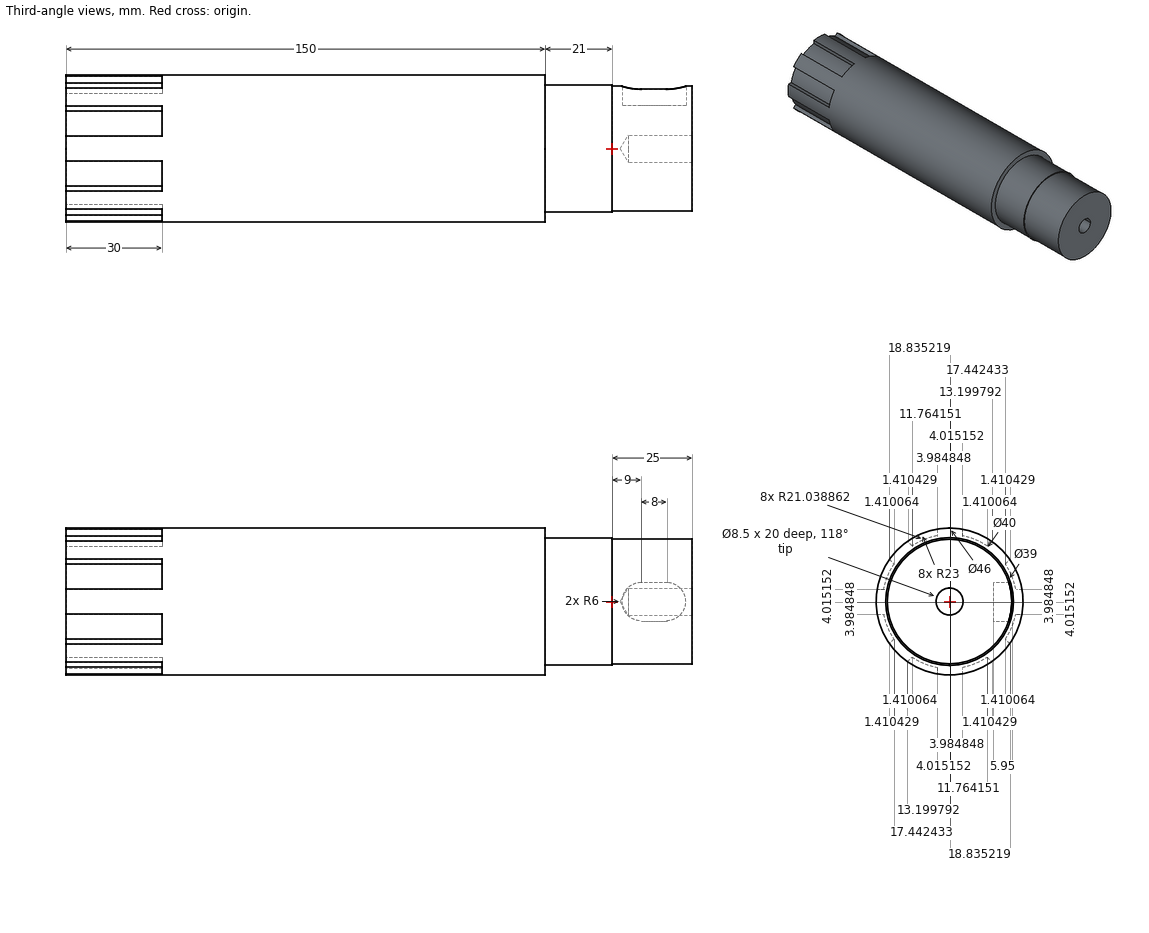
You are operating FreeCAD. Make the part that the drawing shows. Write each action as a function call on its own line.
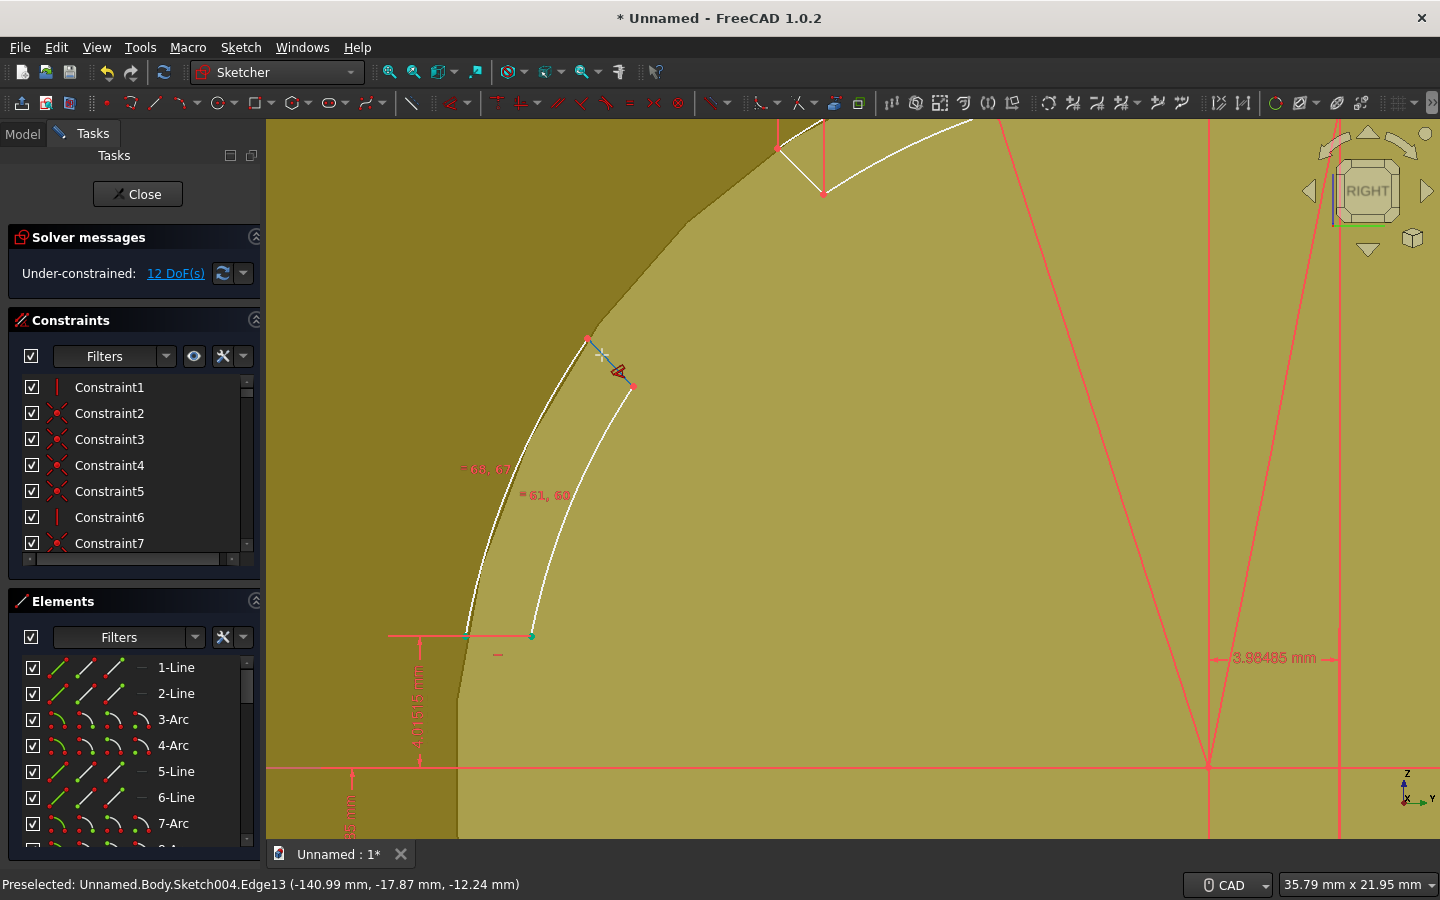
click(602, 353)
click(611, 305)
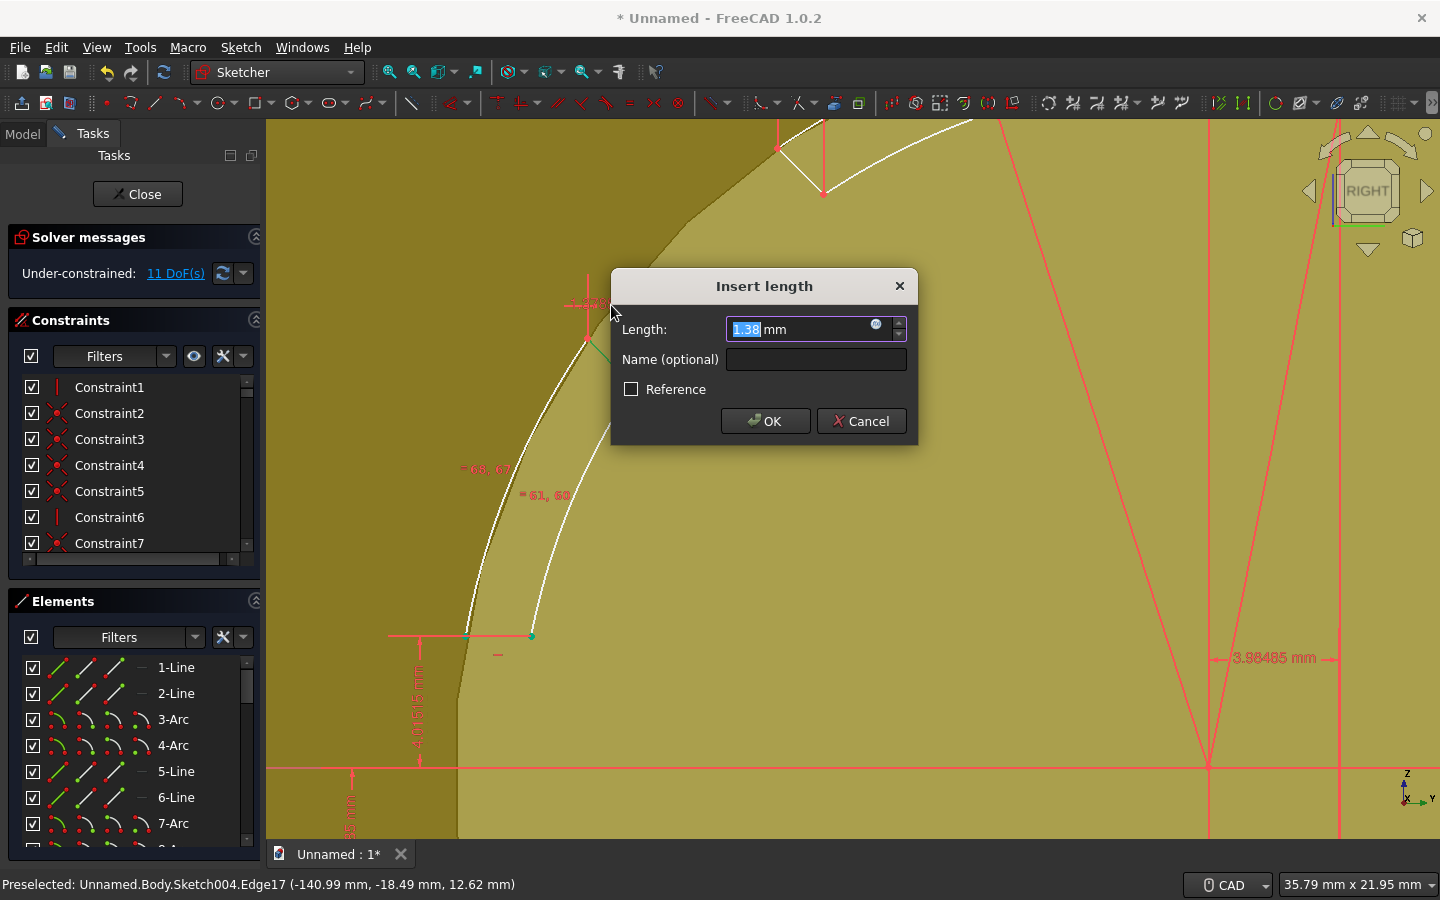
text(1.410064)
key(Return)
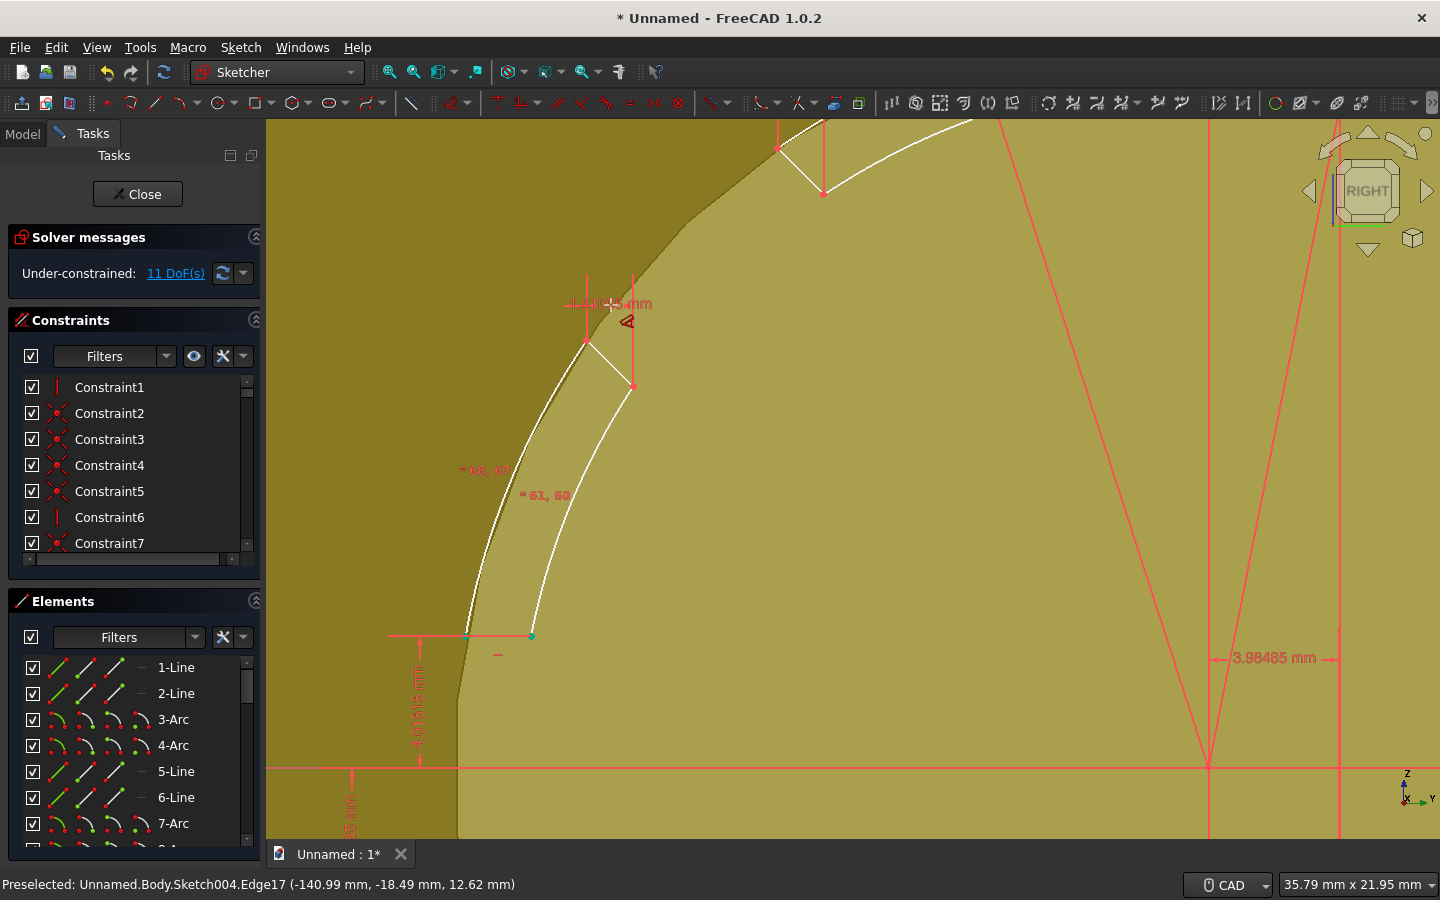
scroll(602, 355, down, 6)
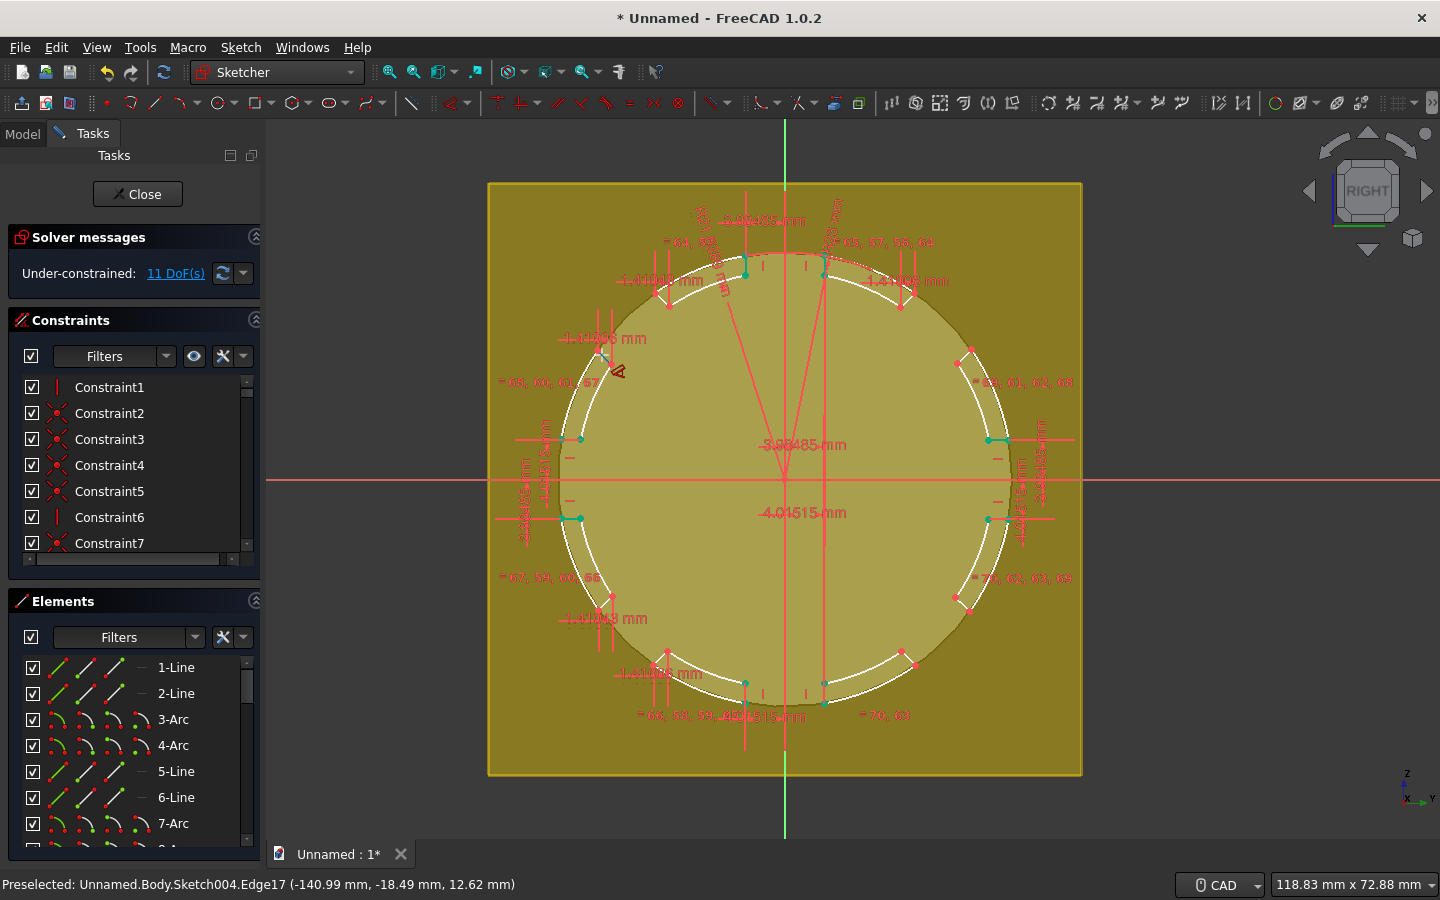
scroll(962, 360, up, 6)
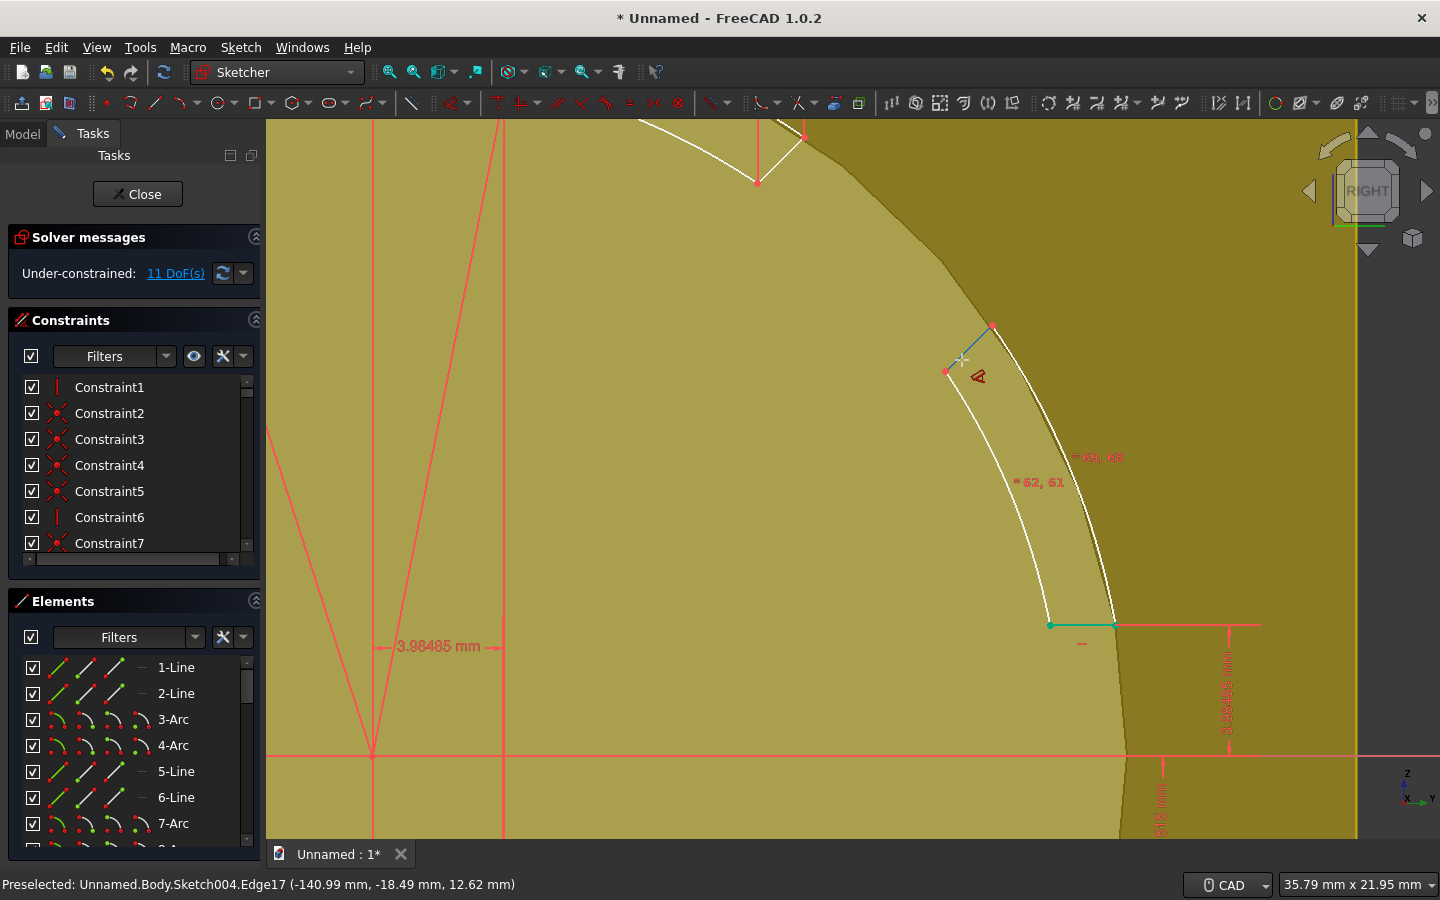
click(960, 358)
click(969, 292)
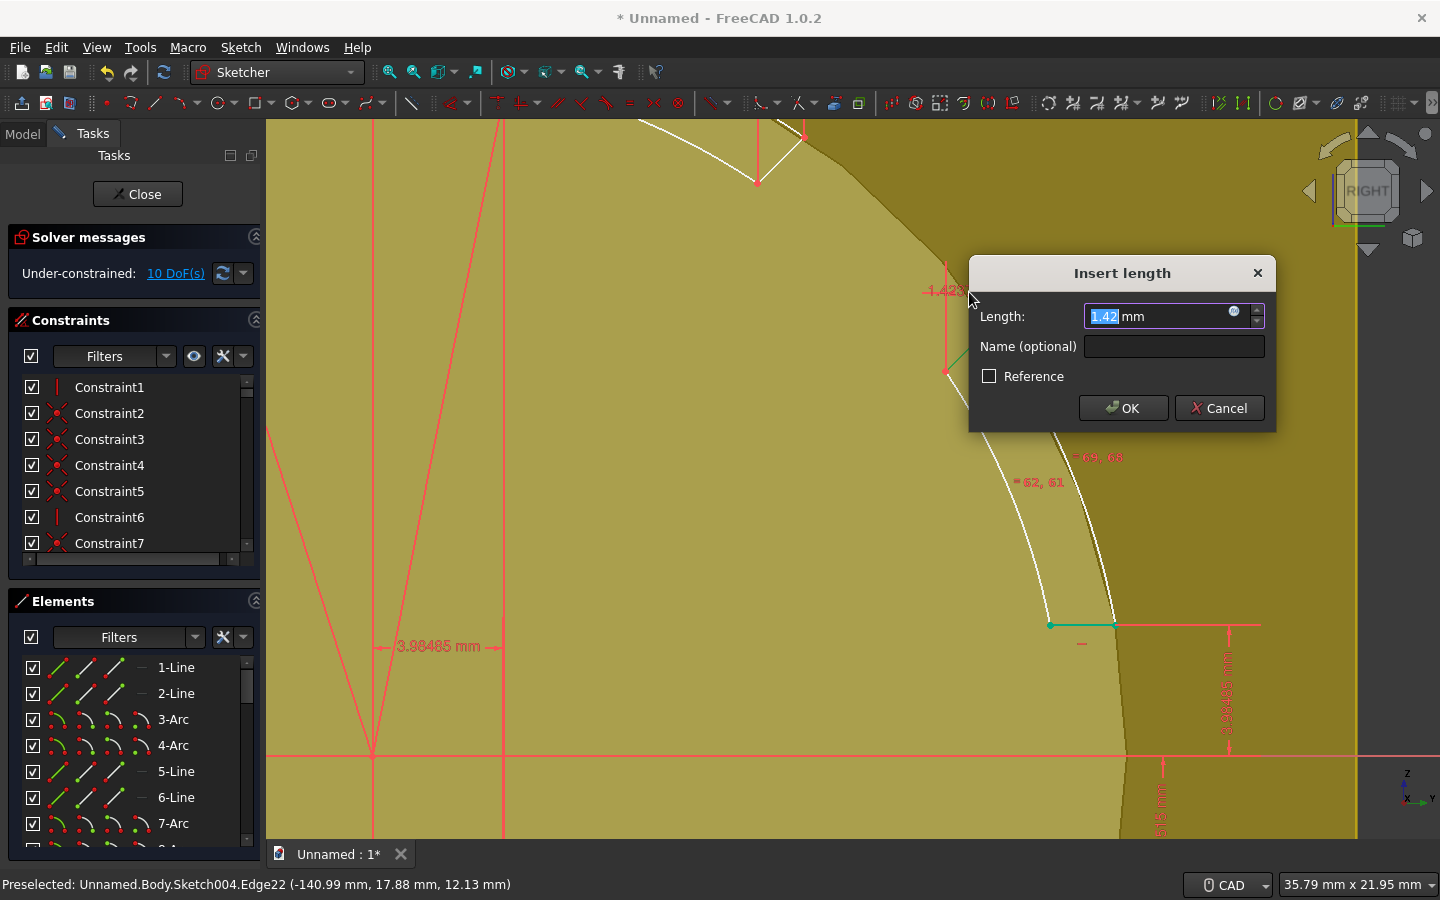
text(1.410429)
key(Return)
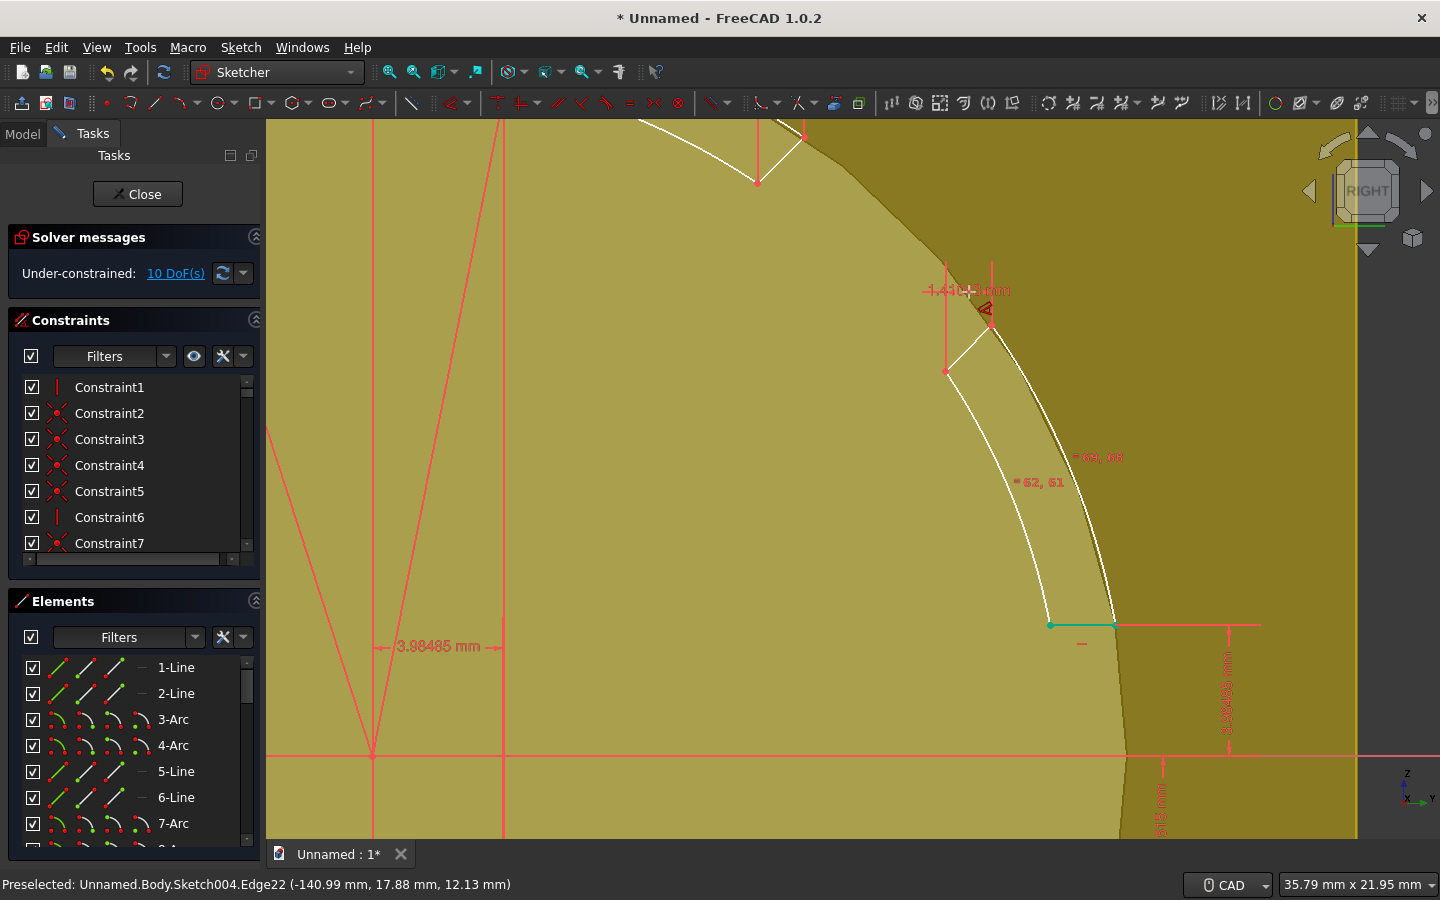
scroll(962, 360, down, 6)